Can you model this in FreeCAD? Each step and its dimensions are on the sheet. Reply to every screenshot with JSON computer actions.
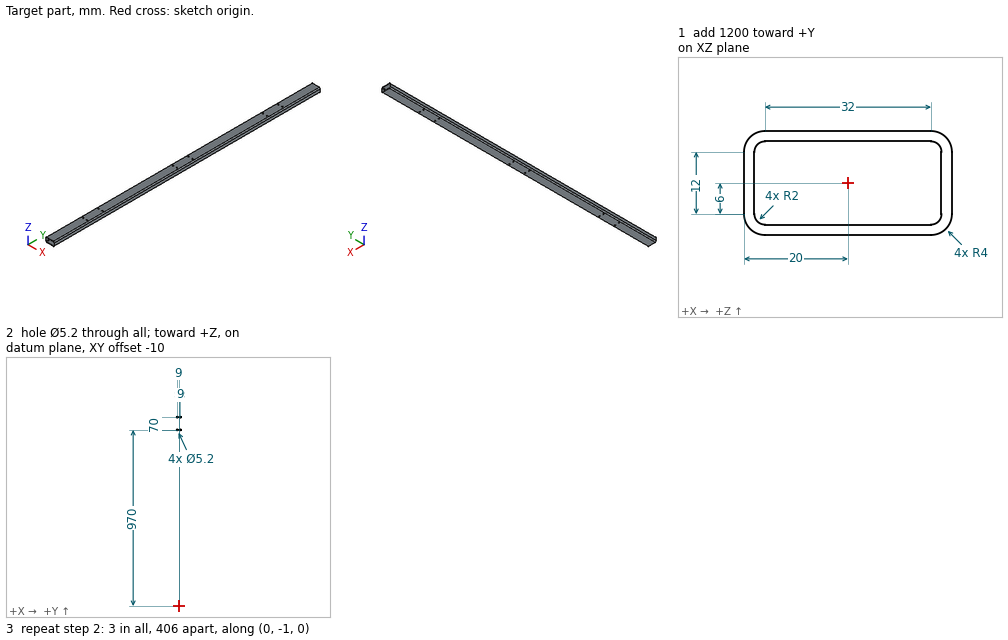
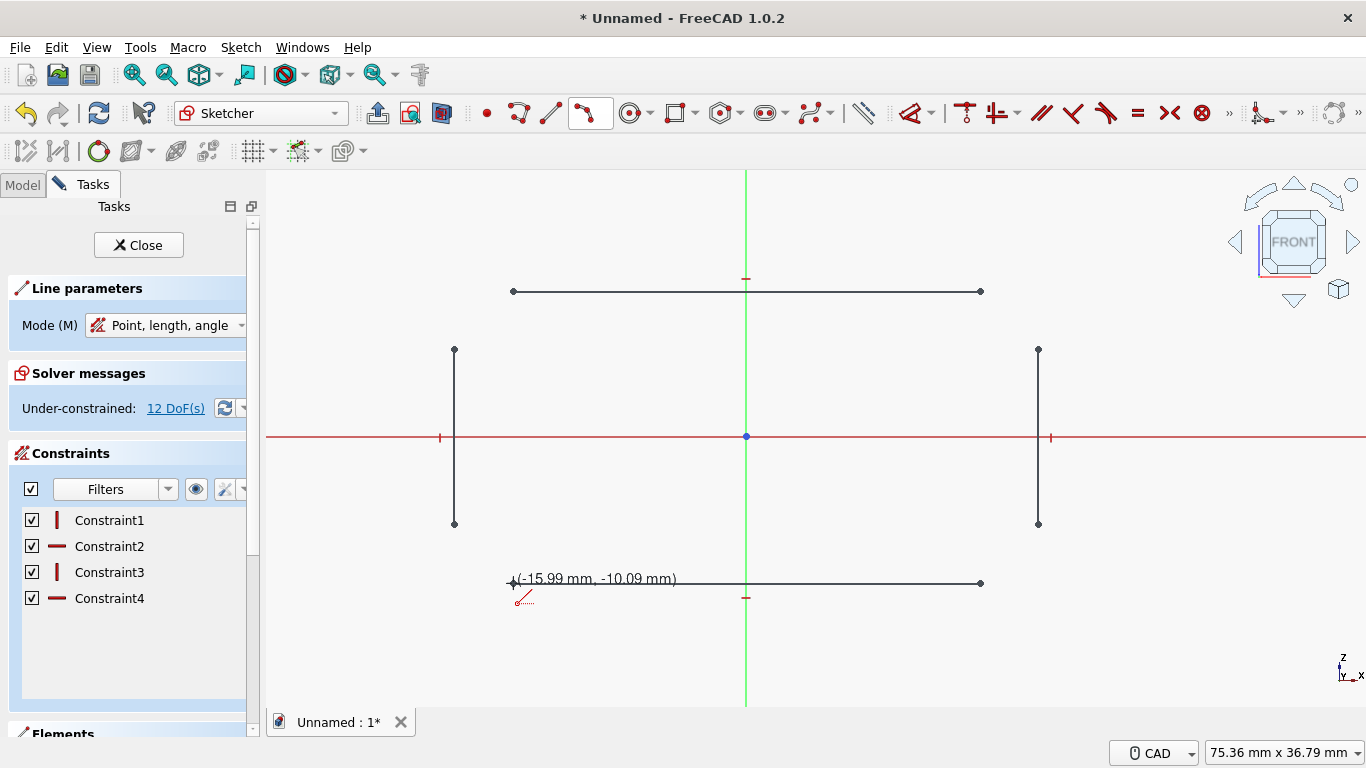
{"action": "left_click", "coordinate": [584, 114]}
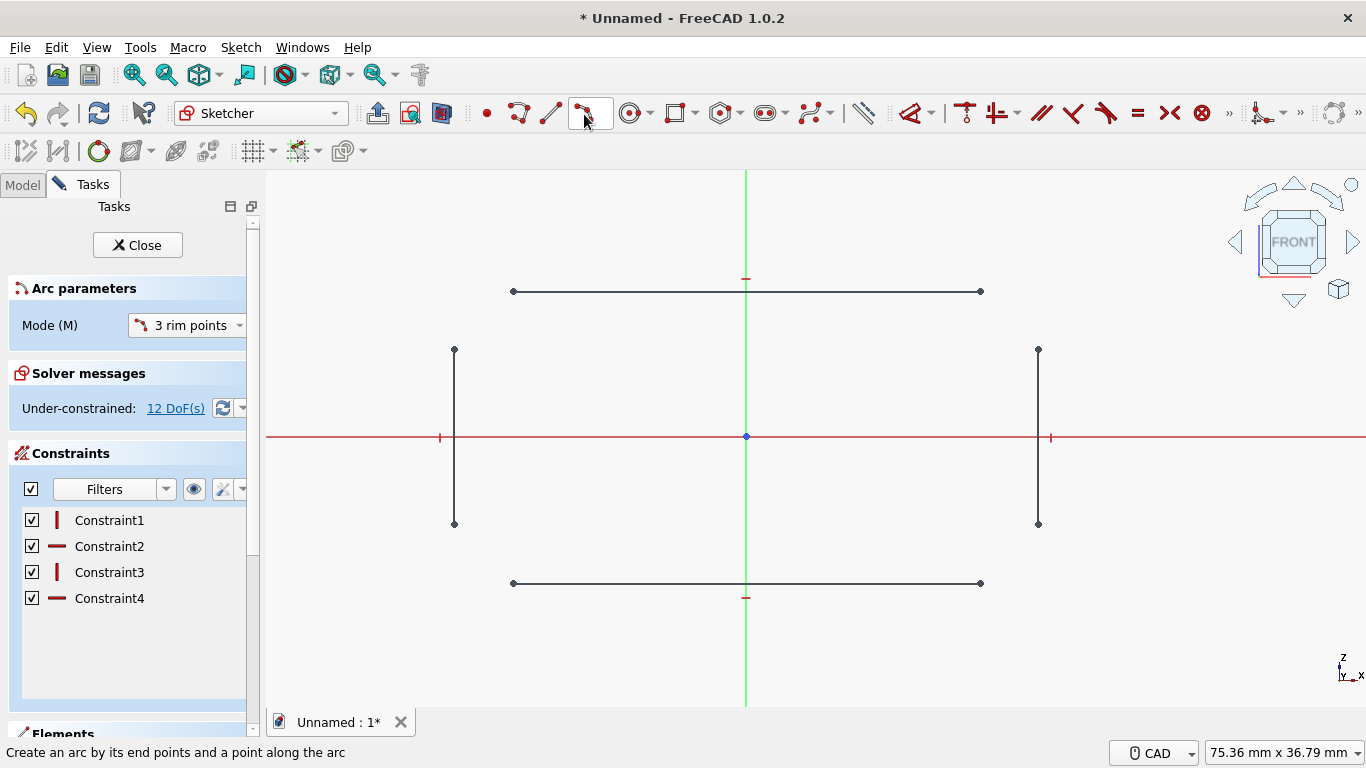
{"action": "left_click", "coordinate": [454, 350]}
{"action": "left_click", "coordinate": [513, 292]}
{"action": "left_click", "coordinate": [472, 308]}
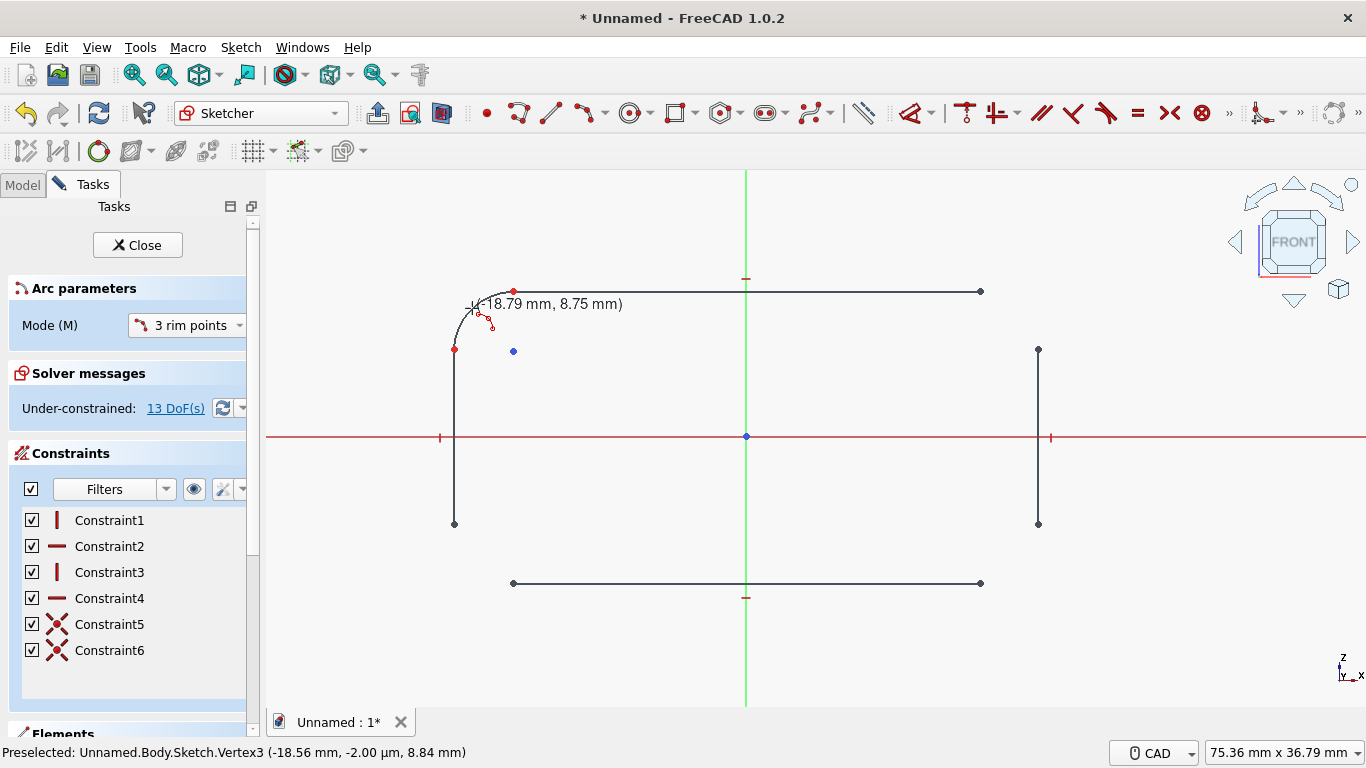
{"action": "left_click", "coordinate": [980, 292]}
{"action": "left_click", "coordinate": [1038, 350]}
{"action": "left_click", "coordinate": [1021, 308]}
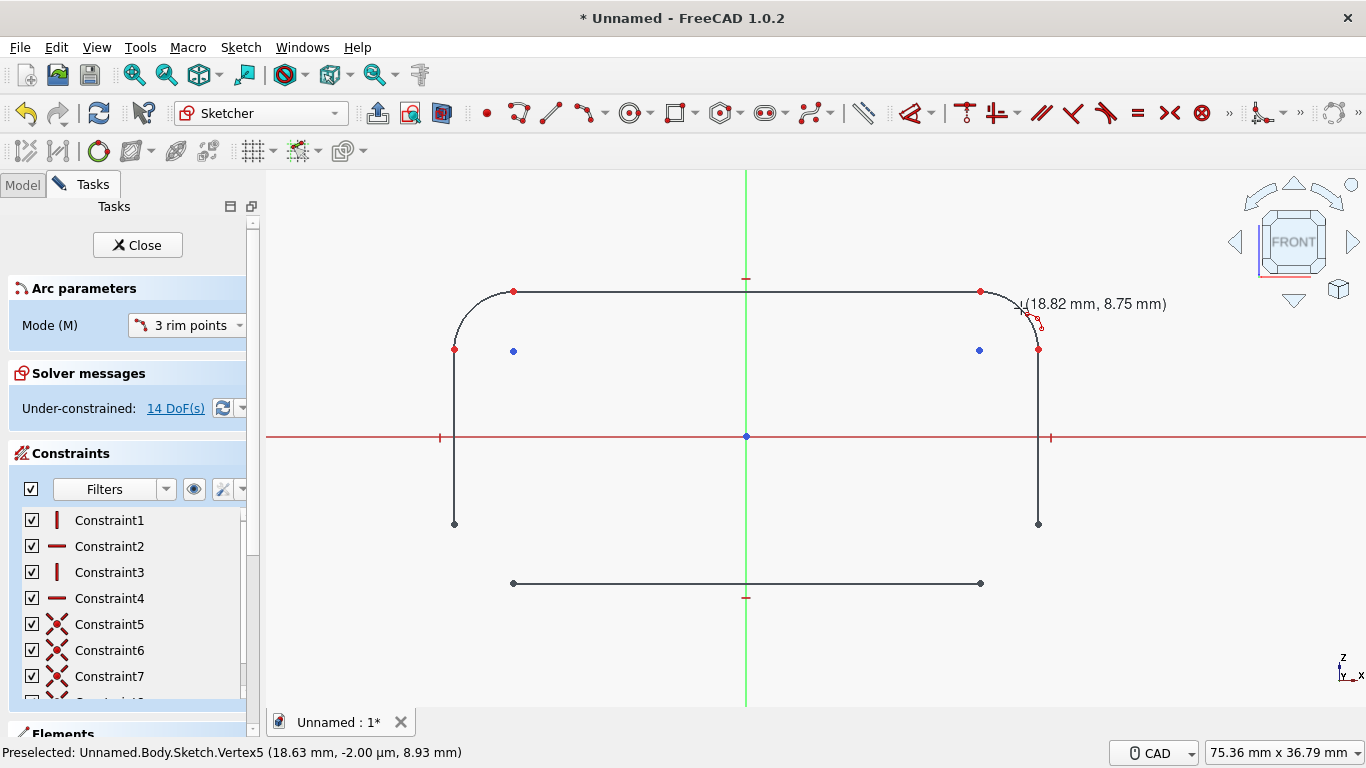
{"action": "left_click", "coordinate": [1038, 525]}
{"action": "left_click", "coordinate": [980, 584]}
{"action": "left_click", "coordinate": [1021, 566]}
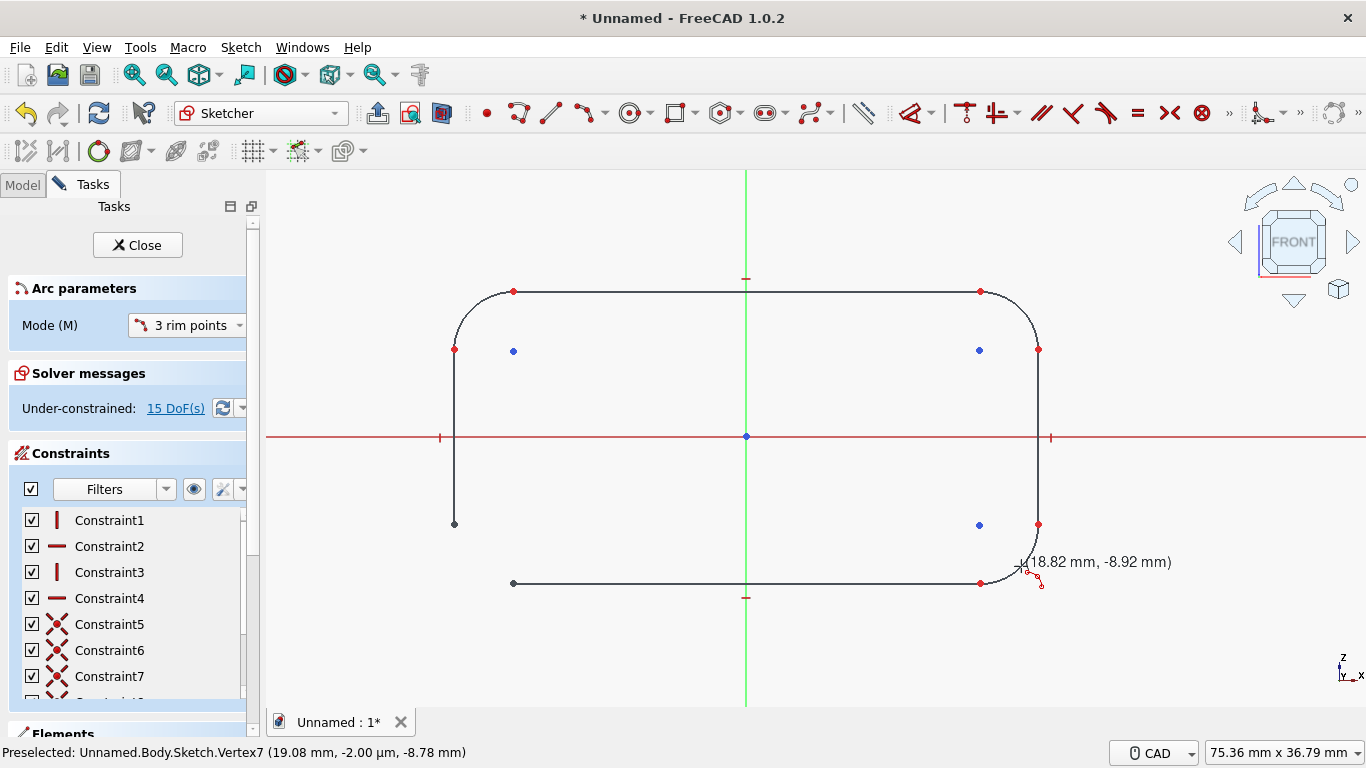
{"action": "left_click", "coordinate": [513, 584]}
{"action": "left_click", "coordinate": [454, 525]}
{"action": "left_click", "coordinate": [472, 566]}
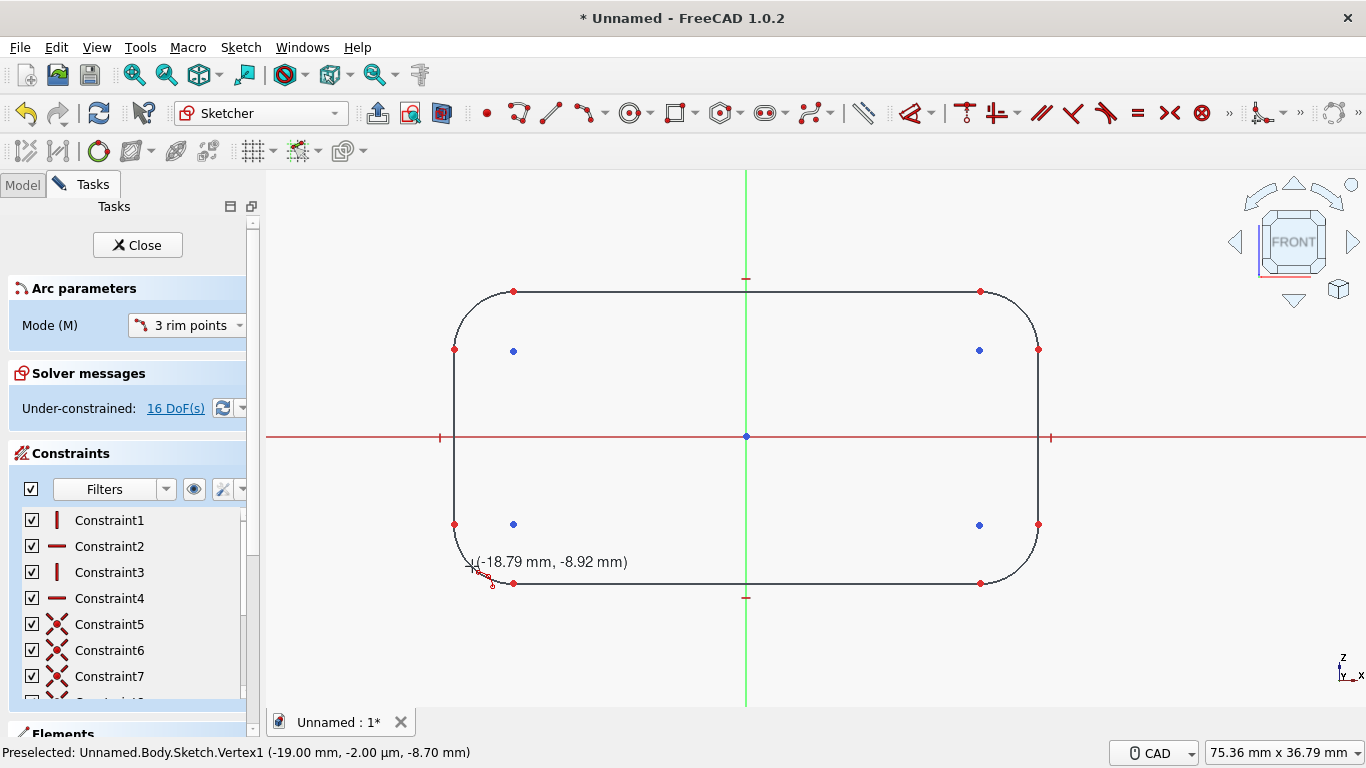
{"action": "key", "text": "g l"}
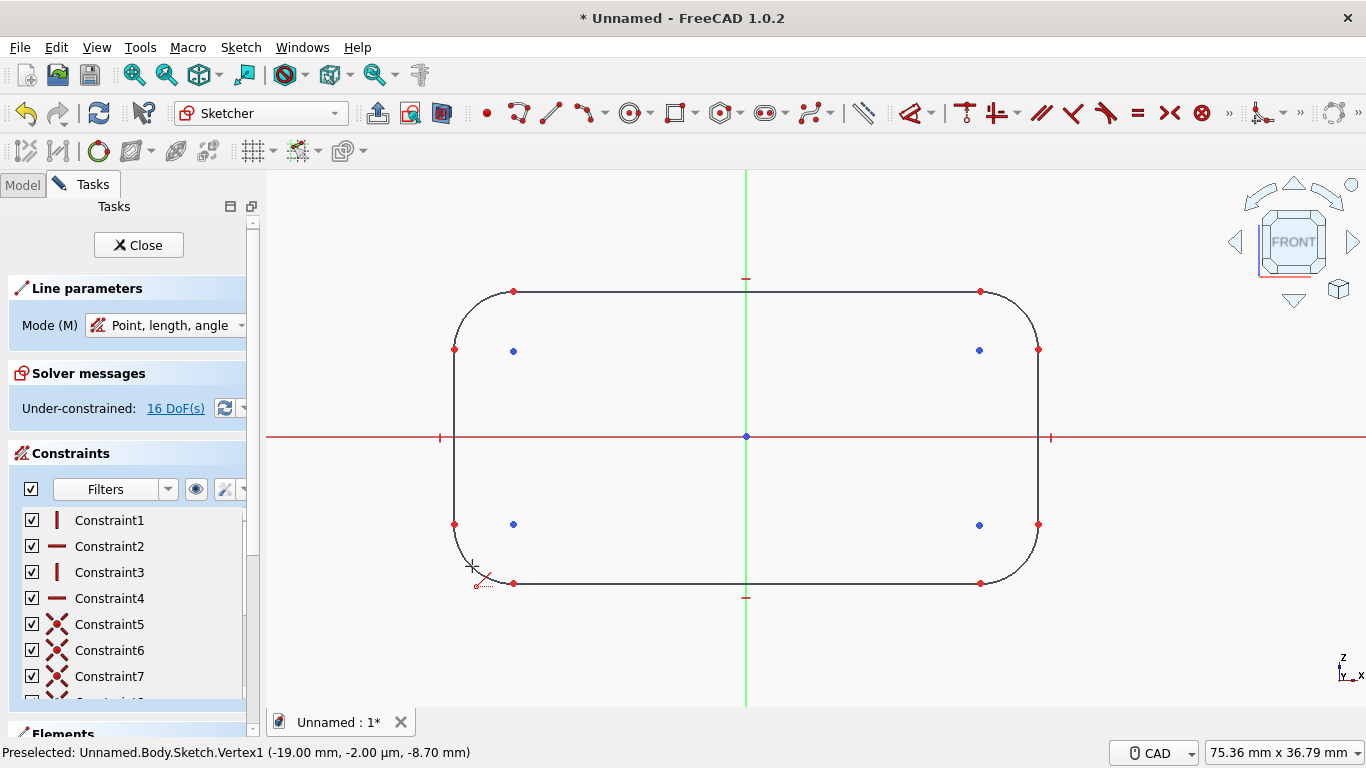
{"action": "left_click", "coordinate": [484, 349]}
{"action": "left_click", "coordinate": [484, 524]}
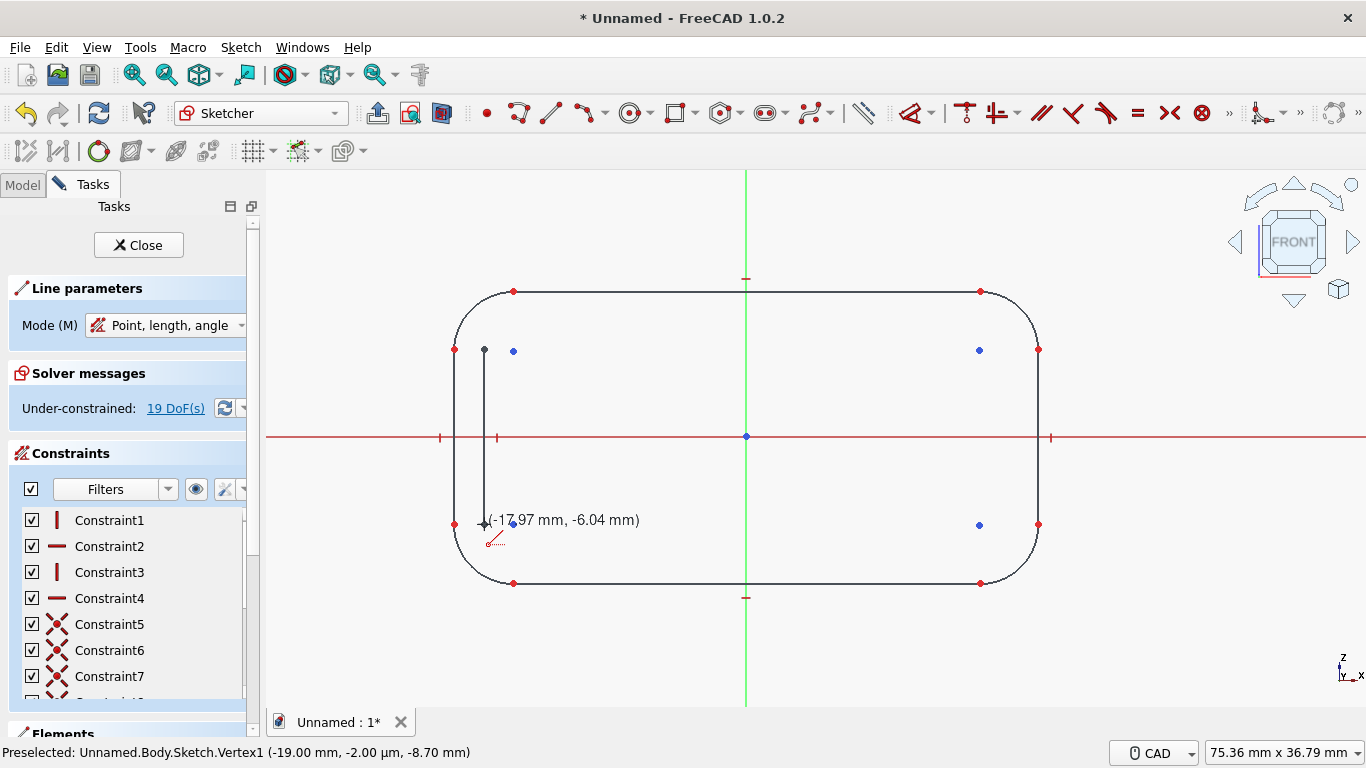
{"action": "left_click", "coordinate": [513, 554]}
{"action": "left_click", "coordinate": [980, 554]}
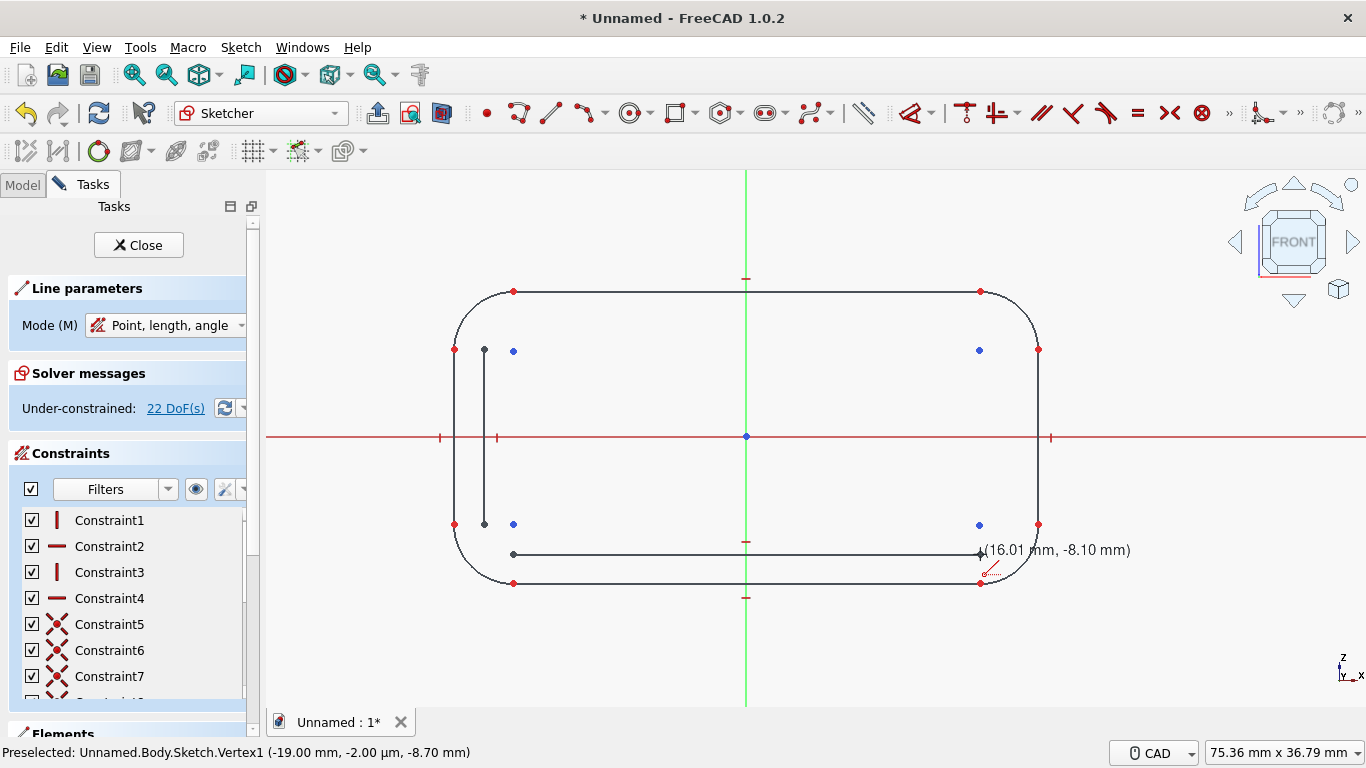
{"action": "left_click", "coordinate": [1009, 524]}
{"action": "left_click", "coordinate": [1009, 349]}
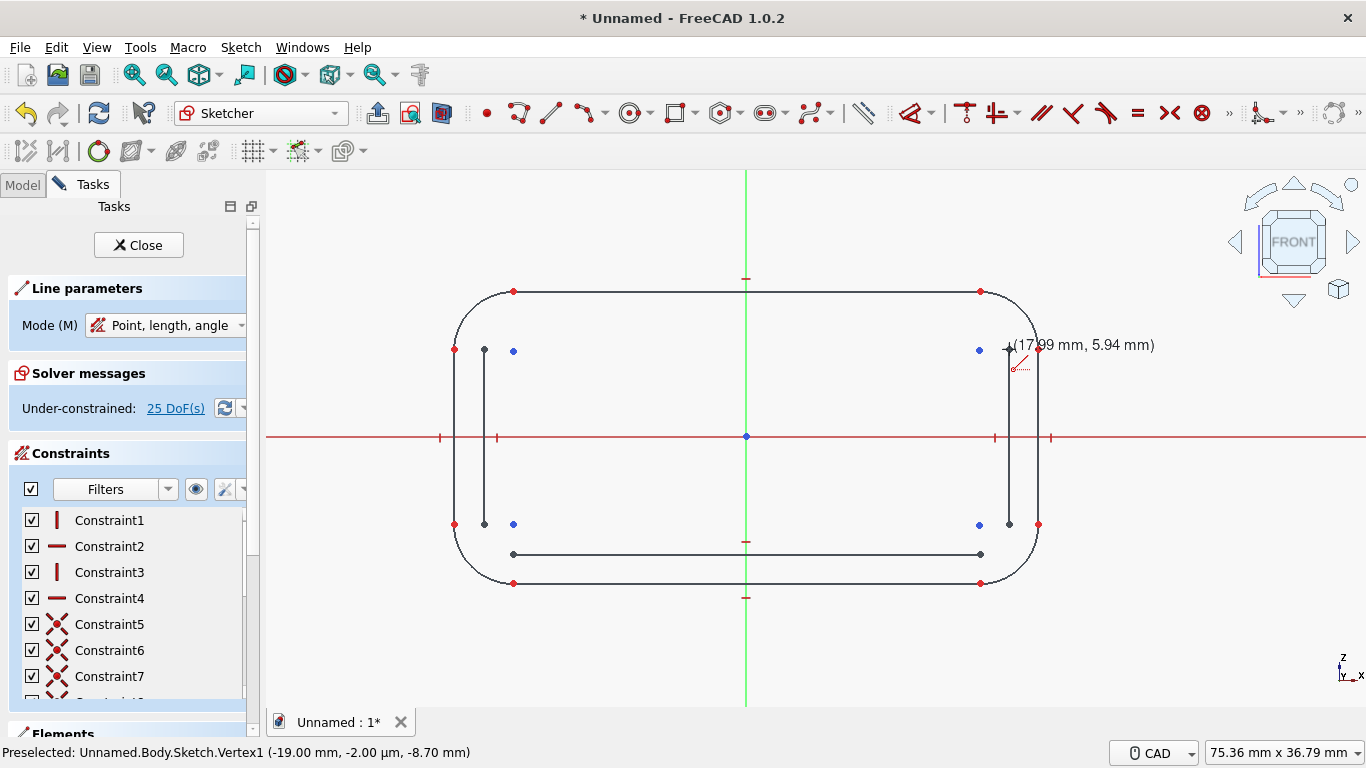
{"action": "left_click", "coordinate": [980, 320]}
{"action": "left_click", "coordinate": [513, 320]}